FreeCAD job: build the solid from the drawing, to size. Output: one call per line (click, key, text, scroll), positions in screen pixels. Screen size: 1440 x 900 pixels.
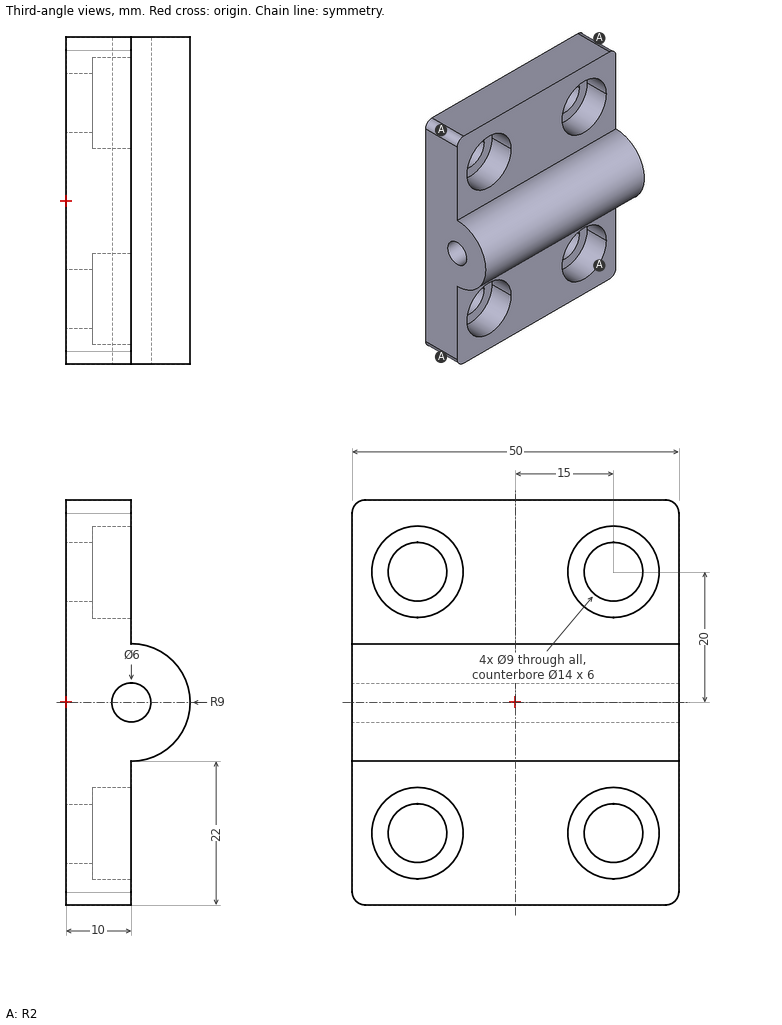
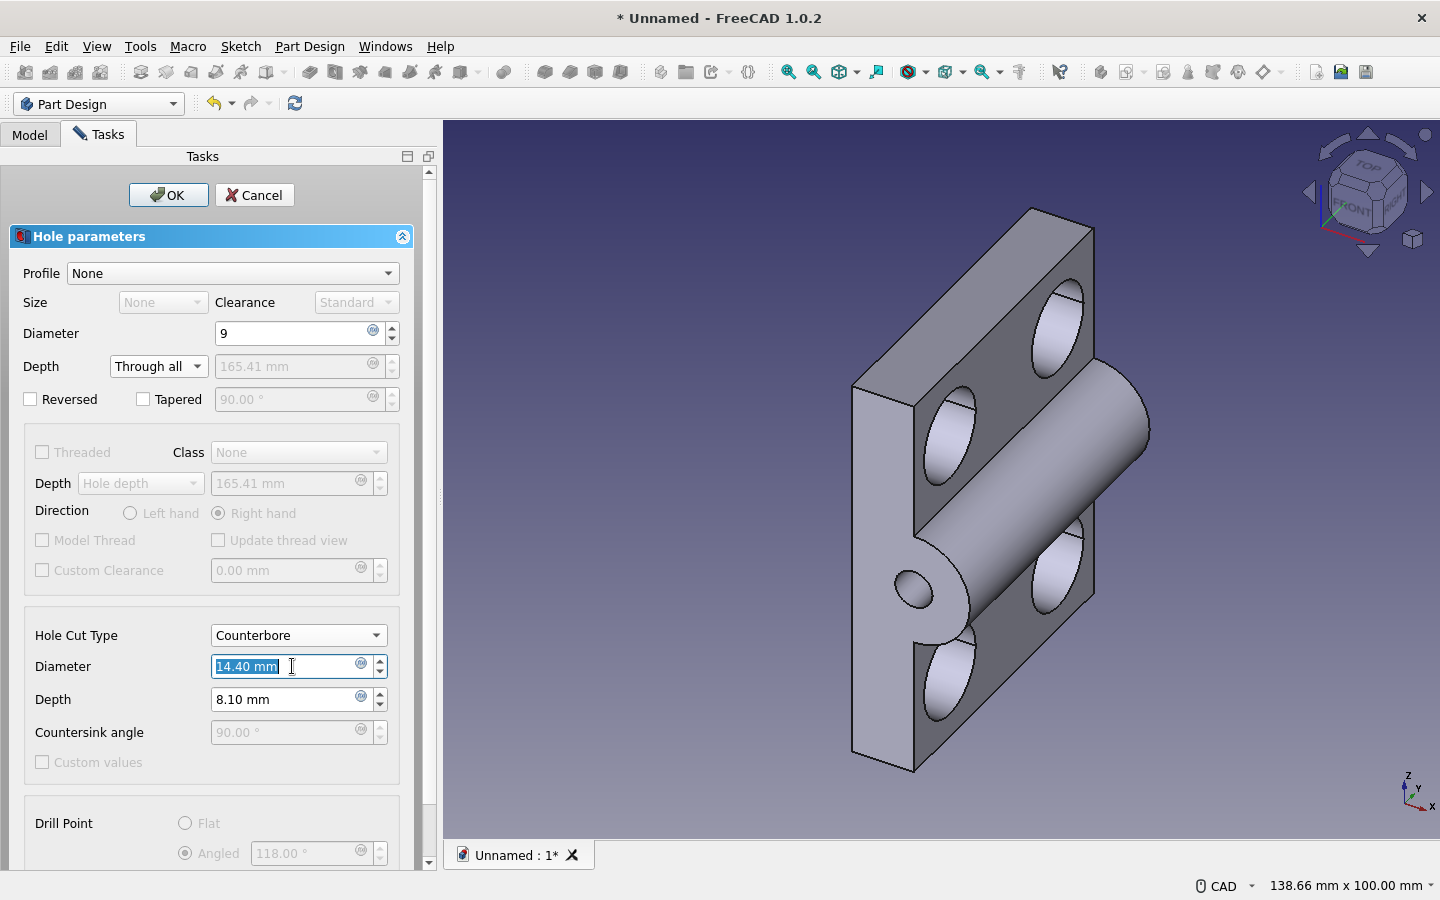
text(14)
key(Tab)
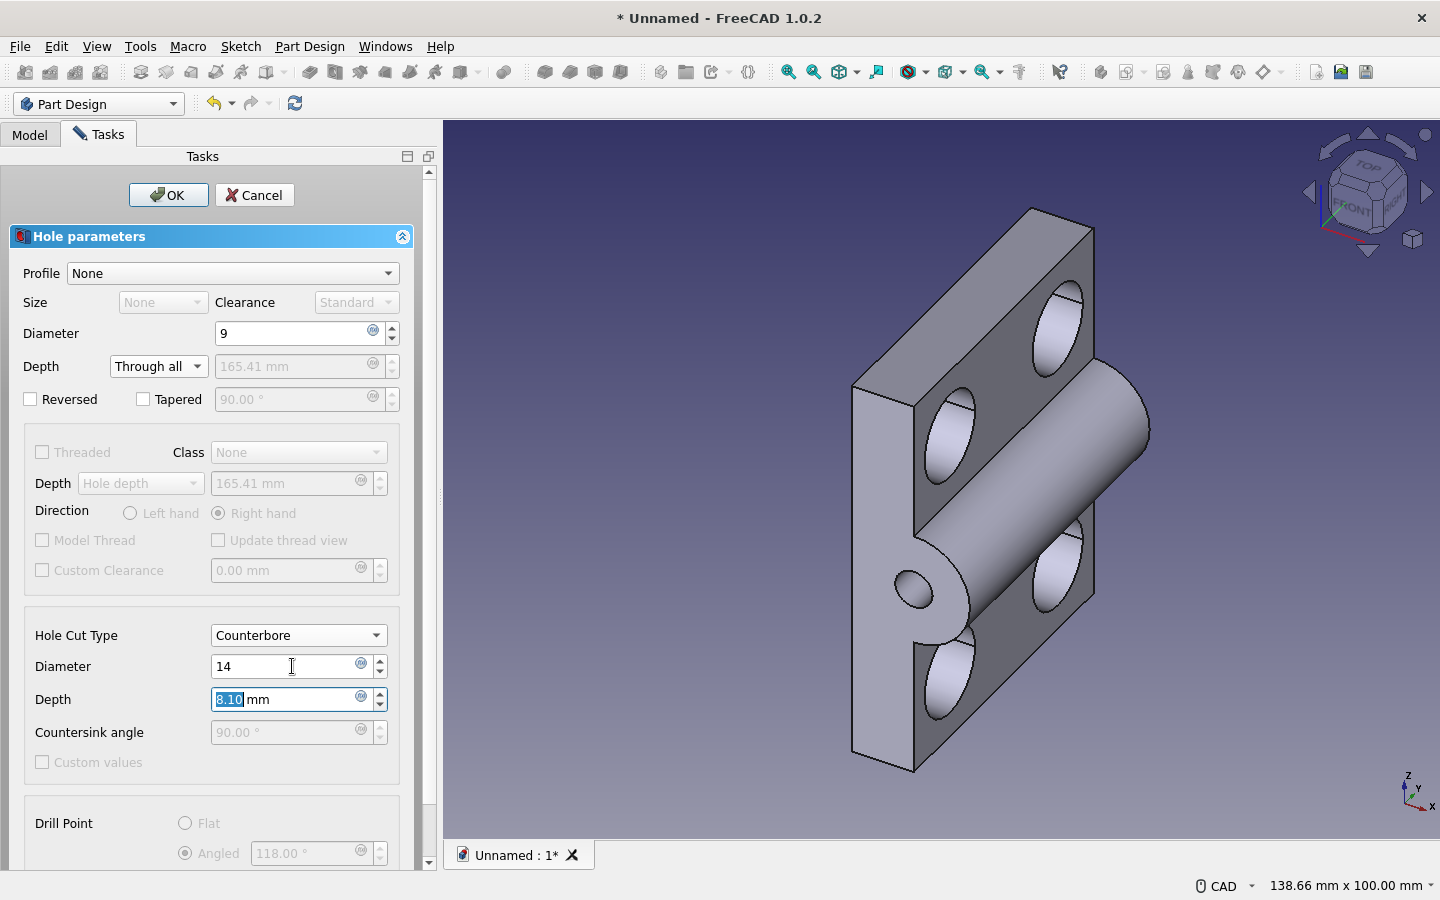
text(6)
key(Tab)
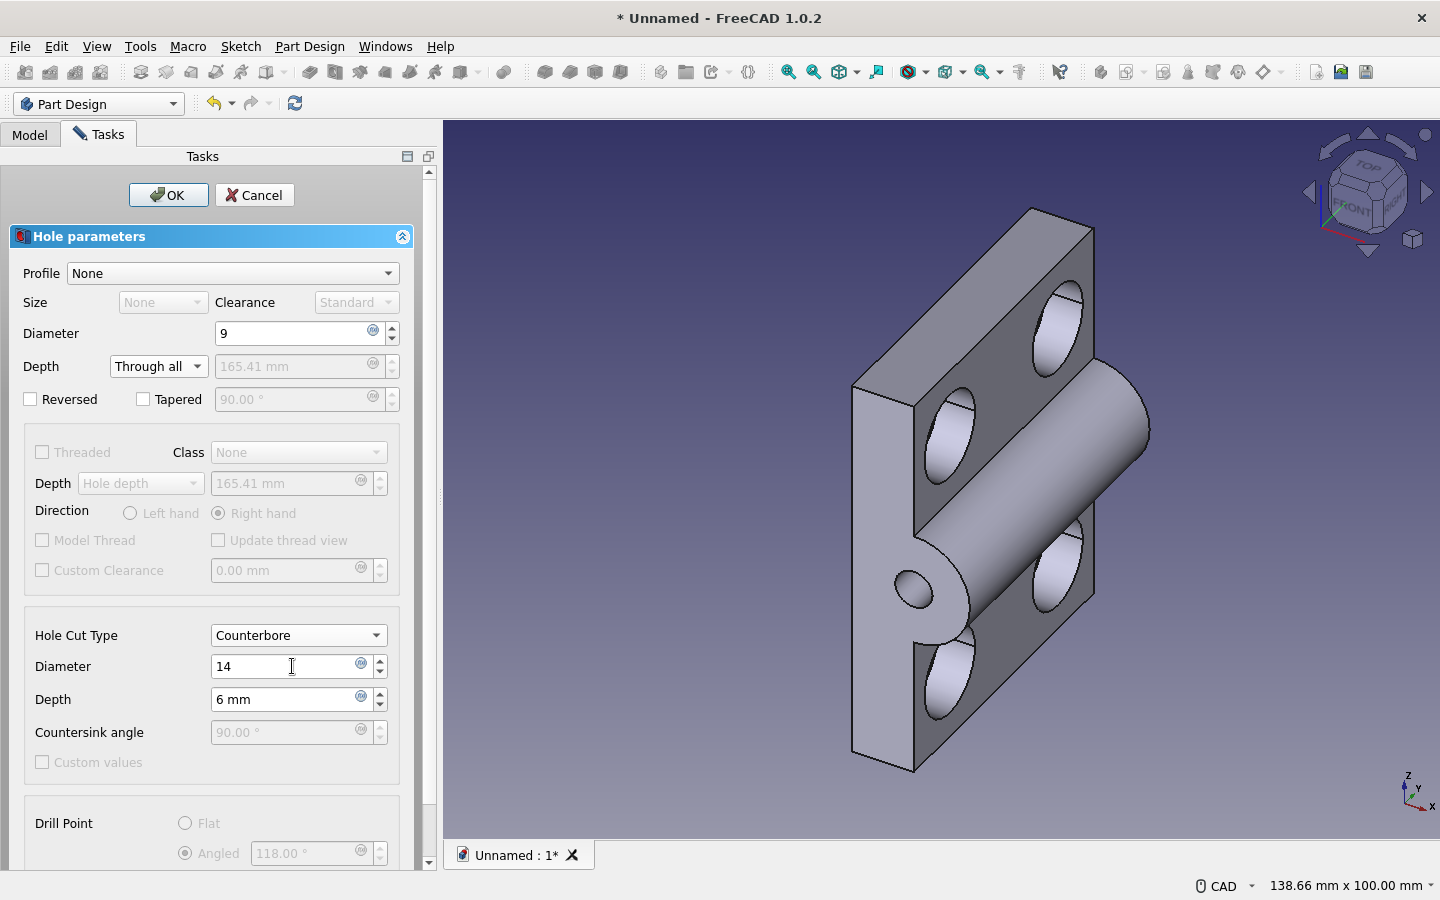
click(169, 195)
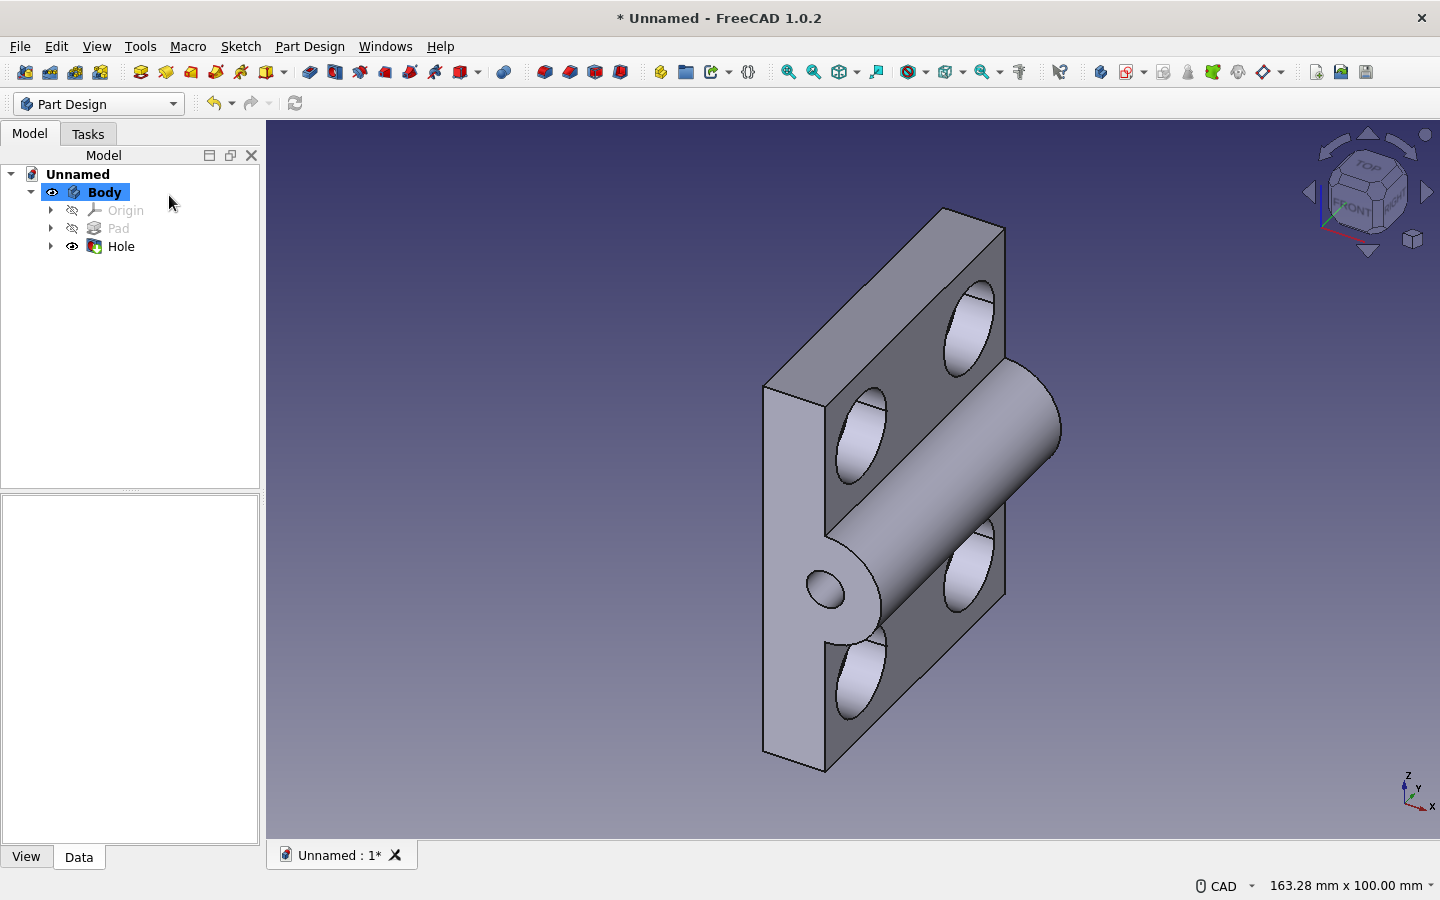
click(794, 396)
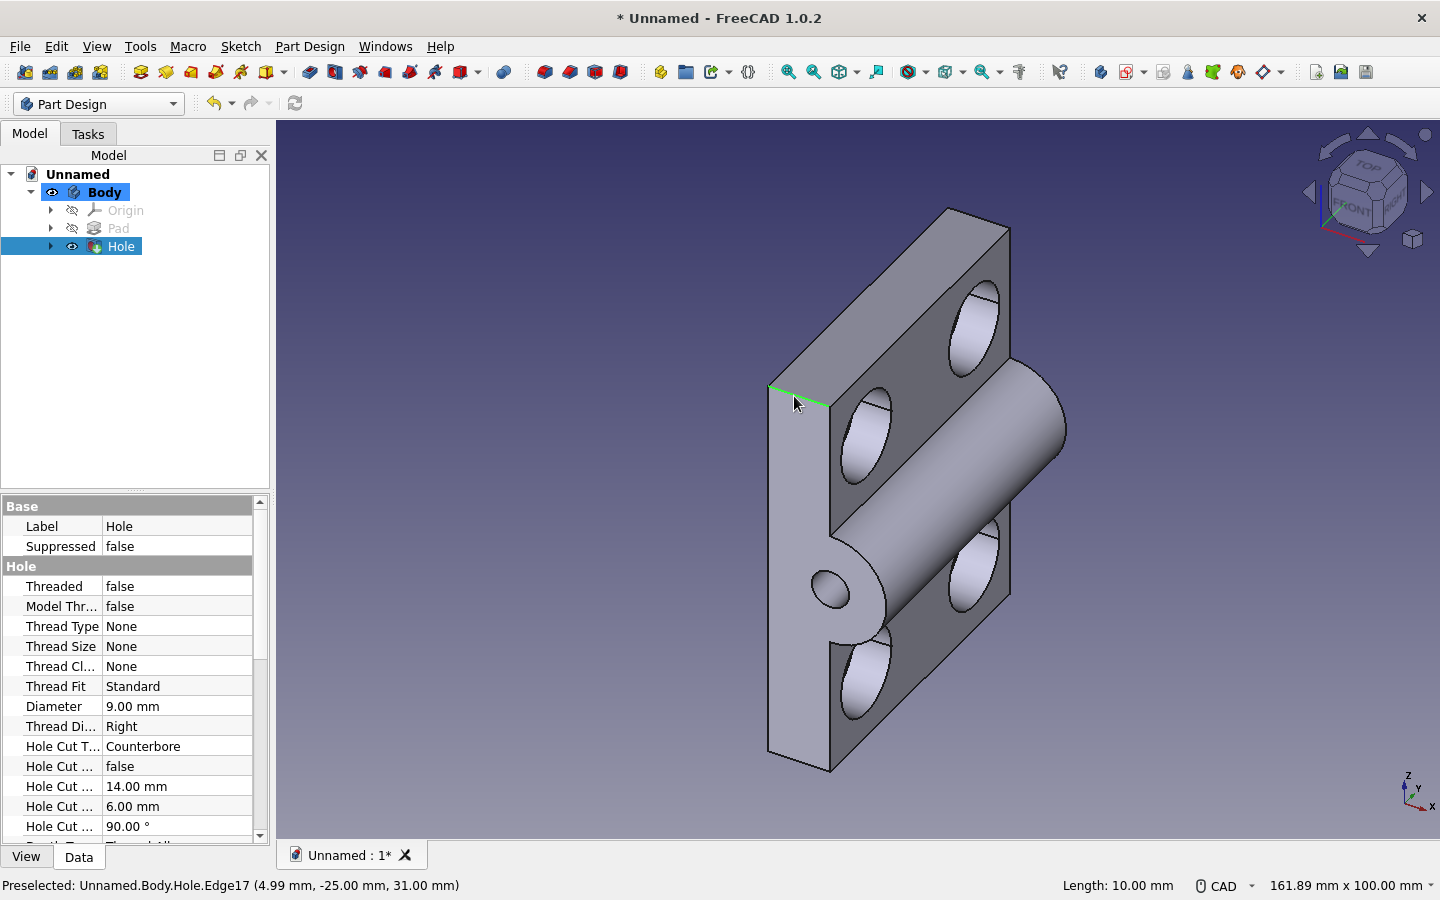
key(0)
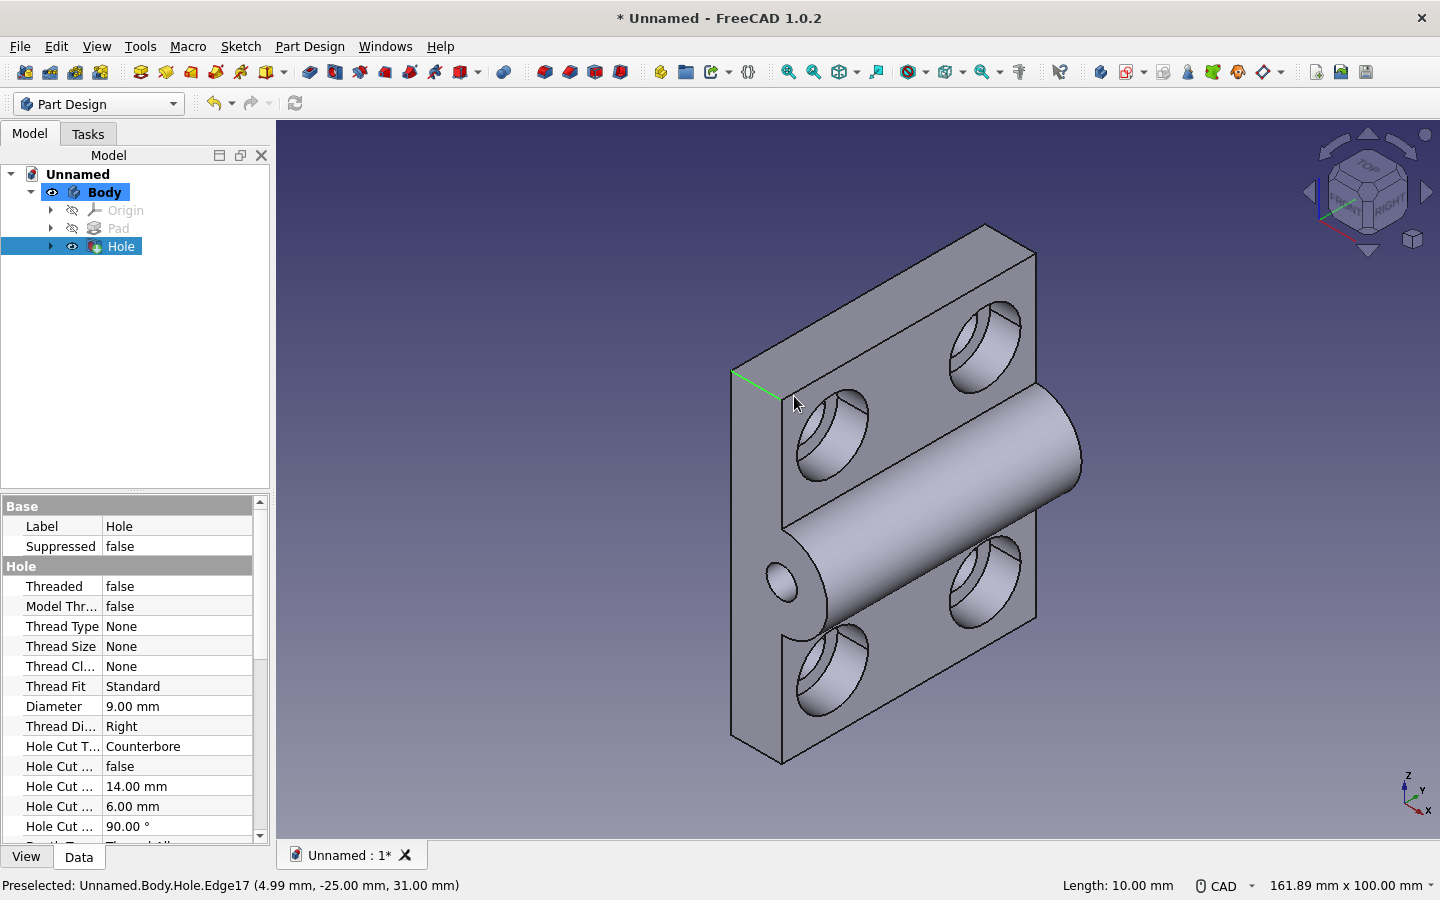
key(2)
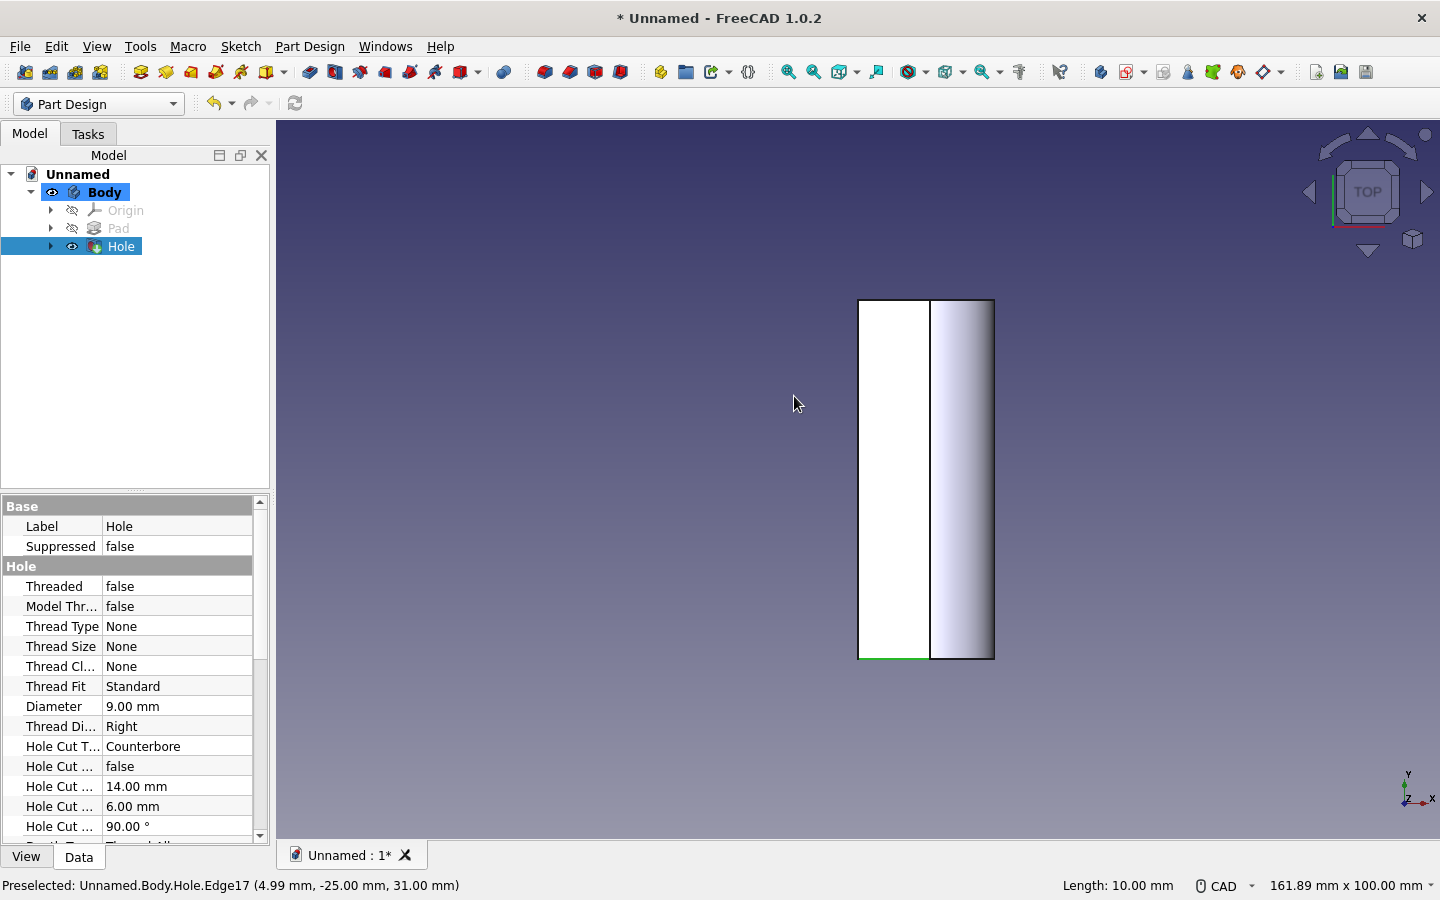
click(894, 299, ctrl)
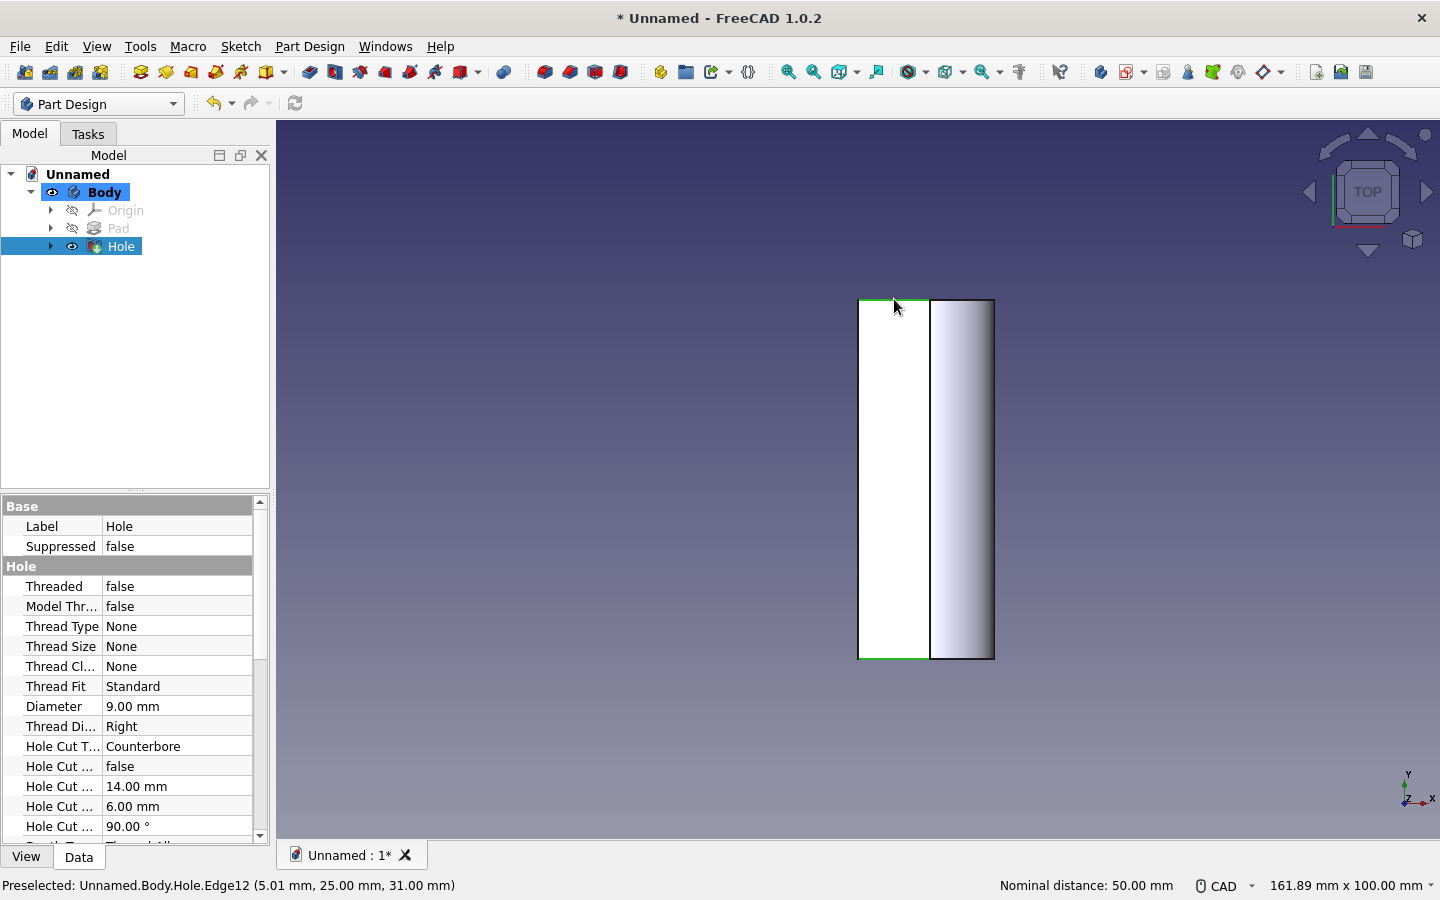
key(1)